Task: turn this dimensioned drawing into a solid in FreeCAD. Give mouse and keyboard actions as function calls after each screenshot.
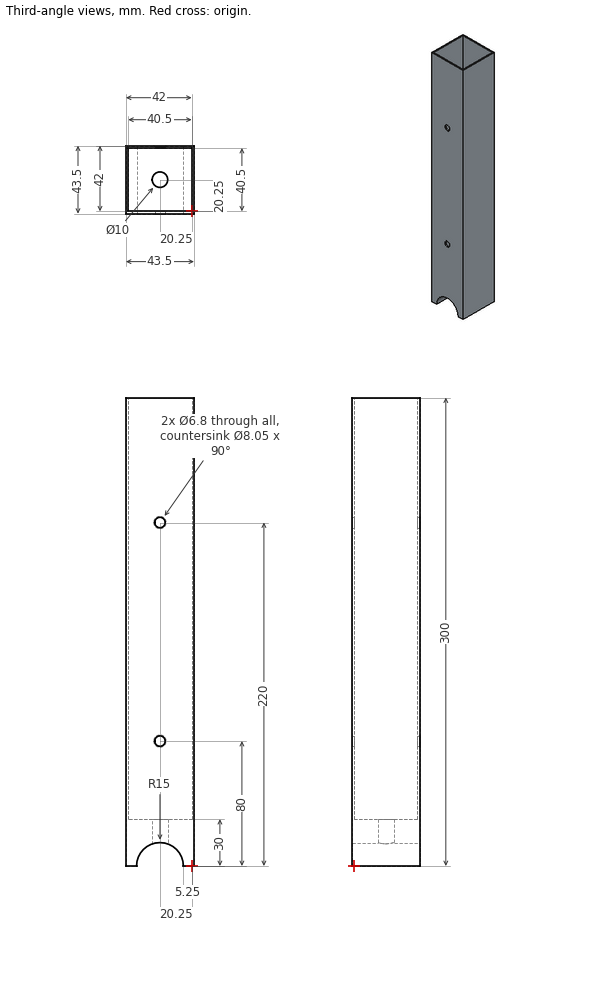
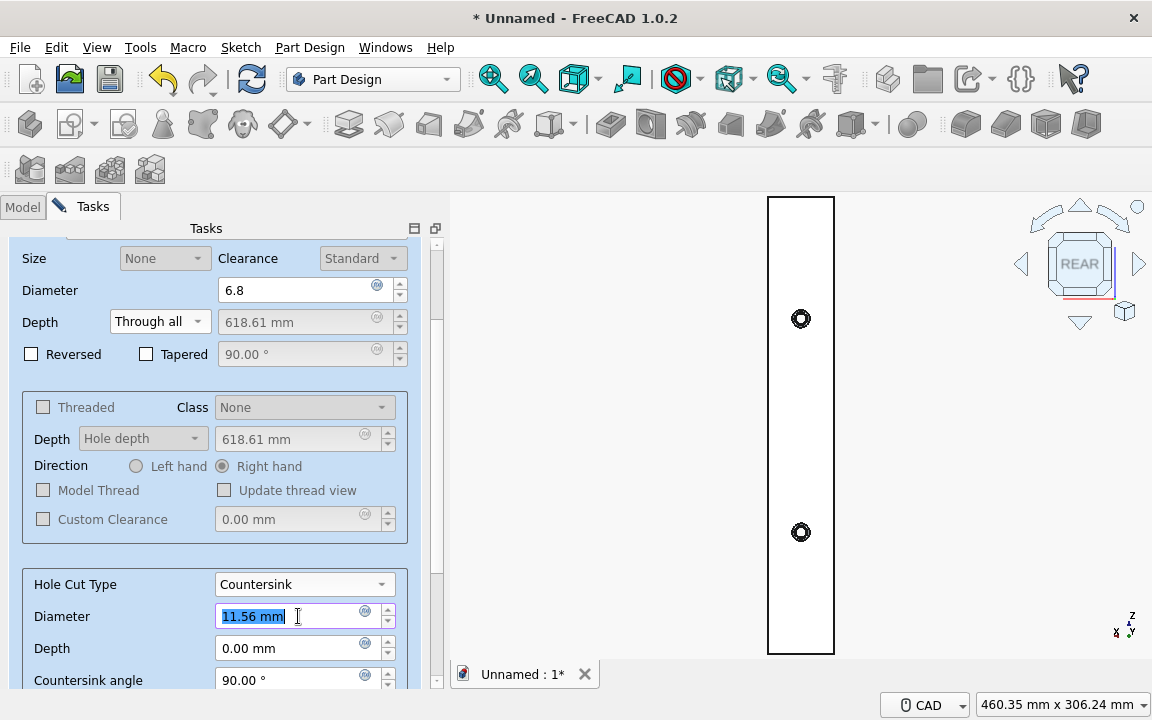
text(8.05)
key(Tab)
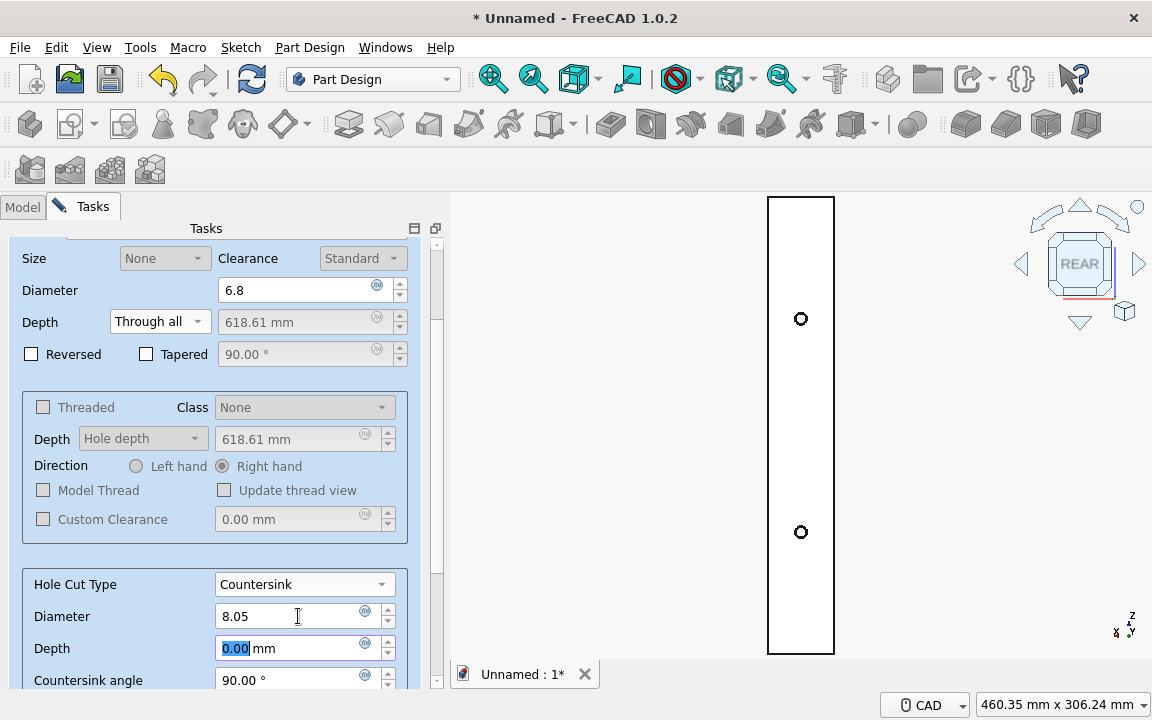
scroll(437, 463, up, 3)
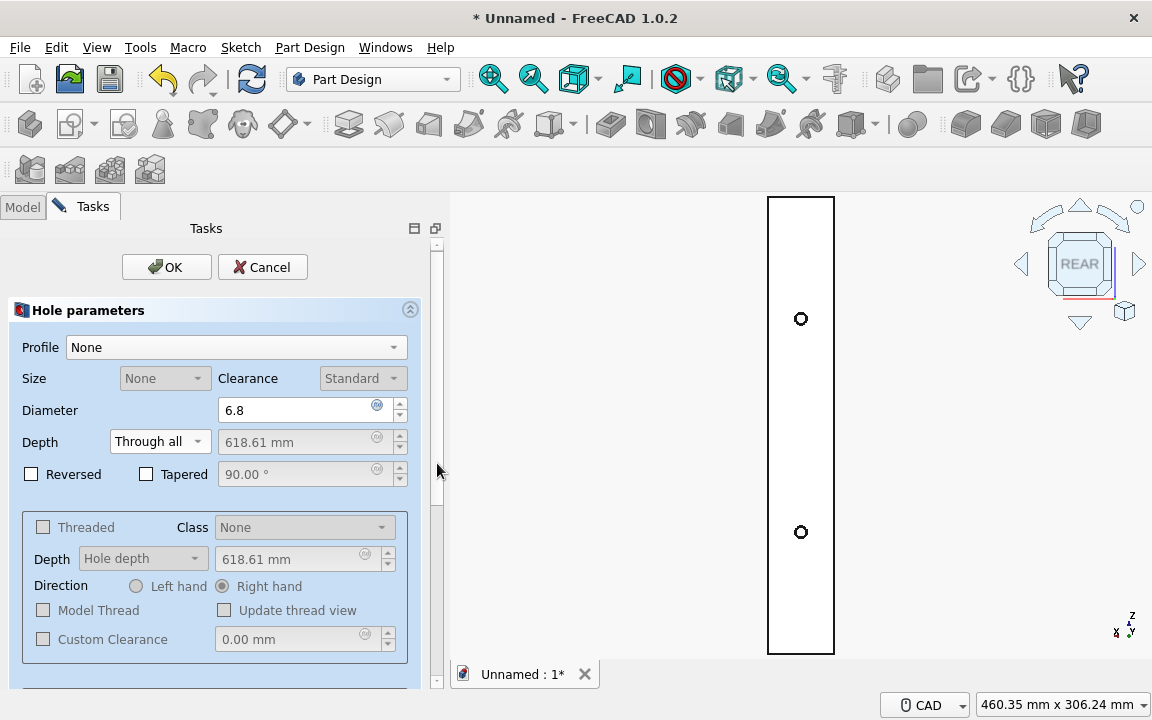
click(167, 267)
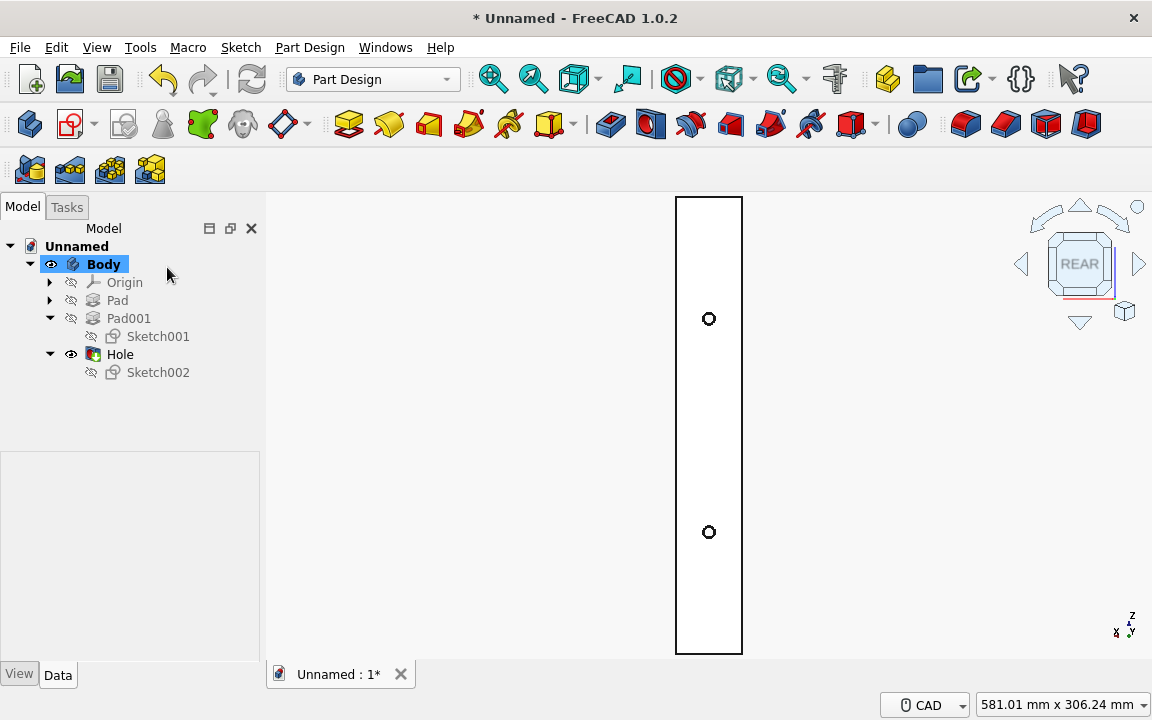
click(709, 359)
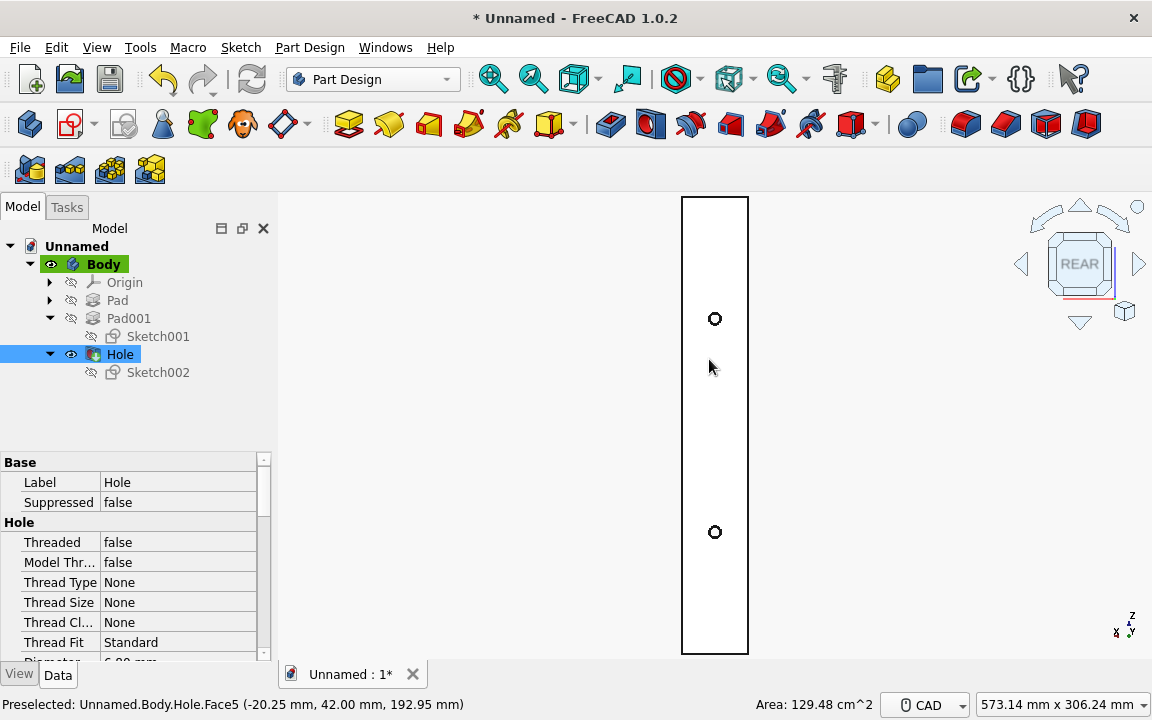
click(70, 124)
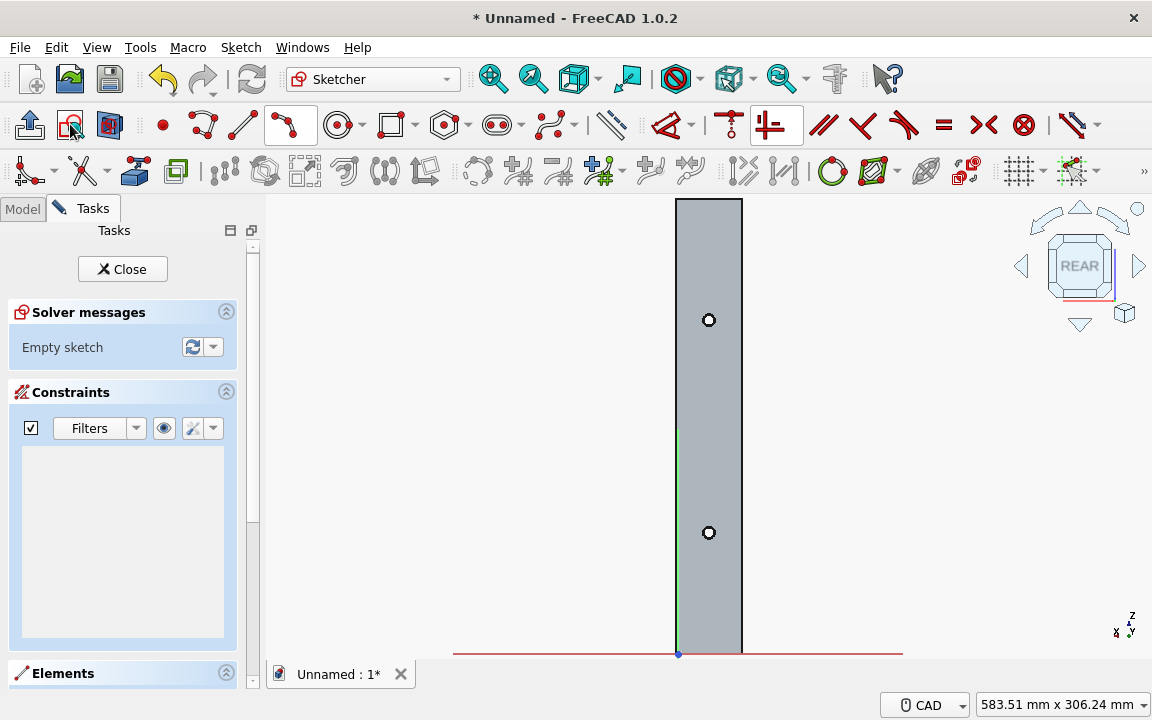
scroll(640, 426, down, 5)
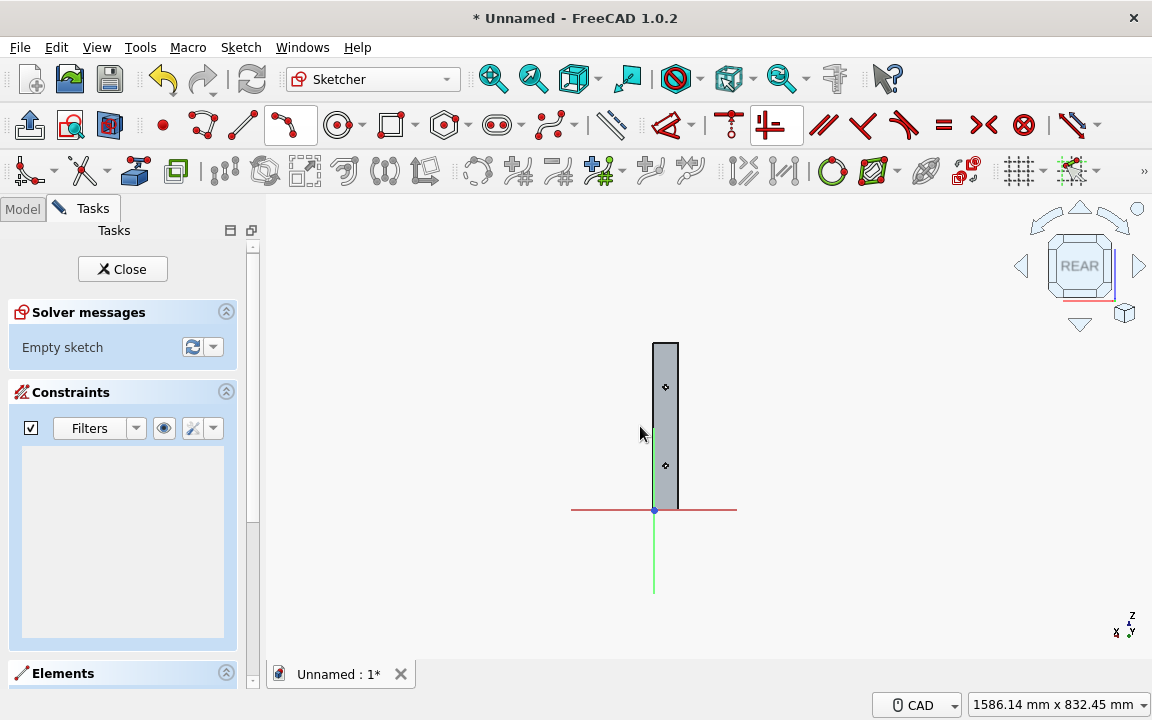
scroll(665, 510, up, 15)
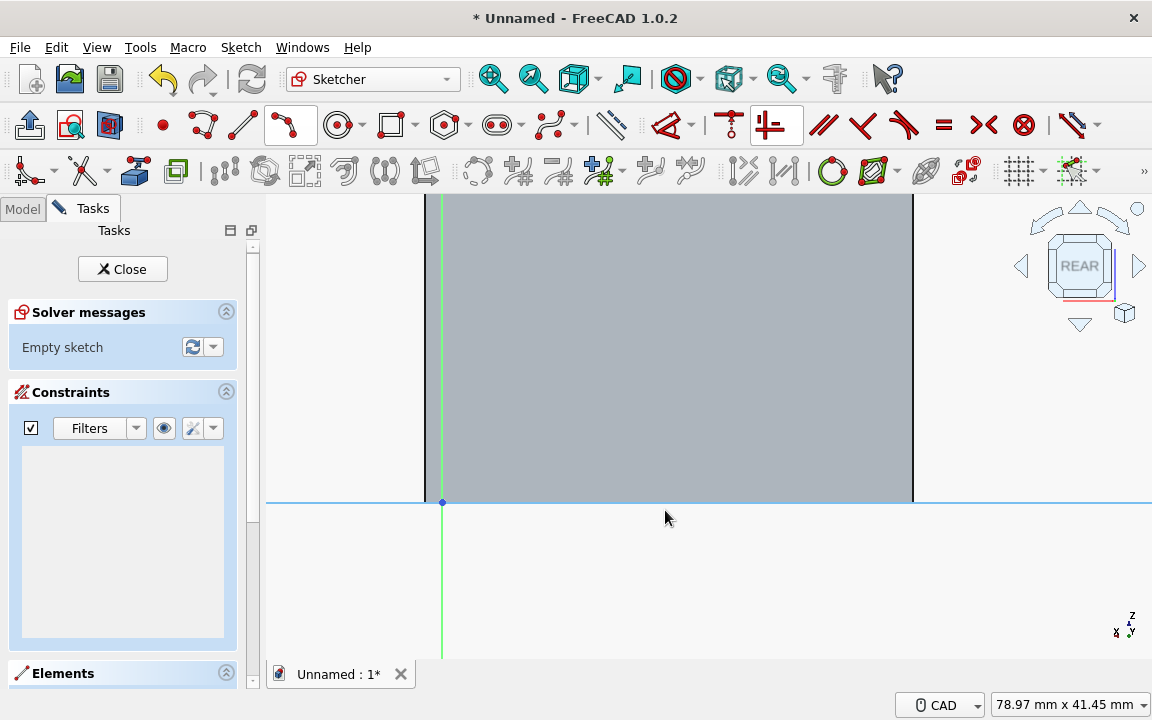
click(244, 126)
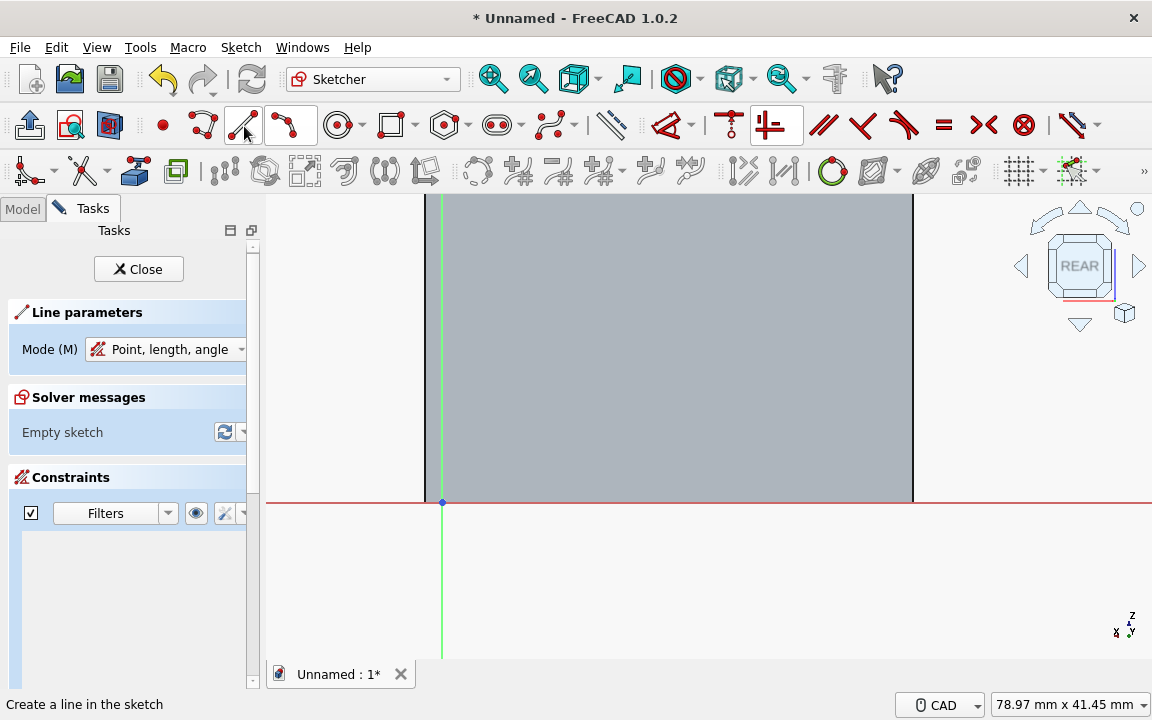
click(501, 503)
click(838, 494)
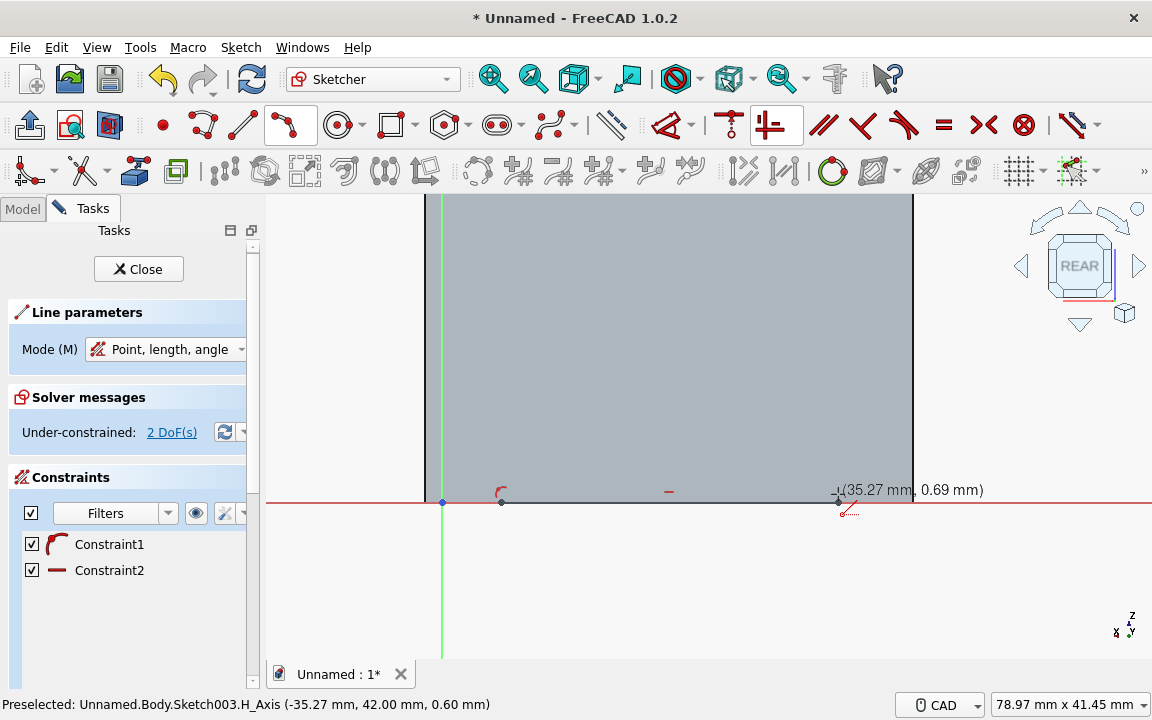
click(284, 126)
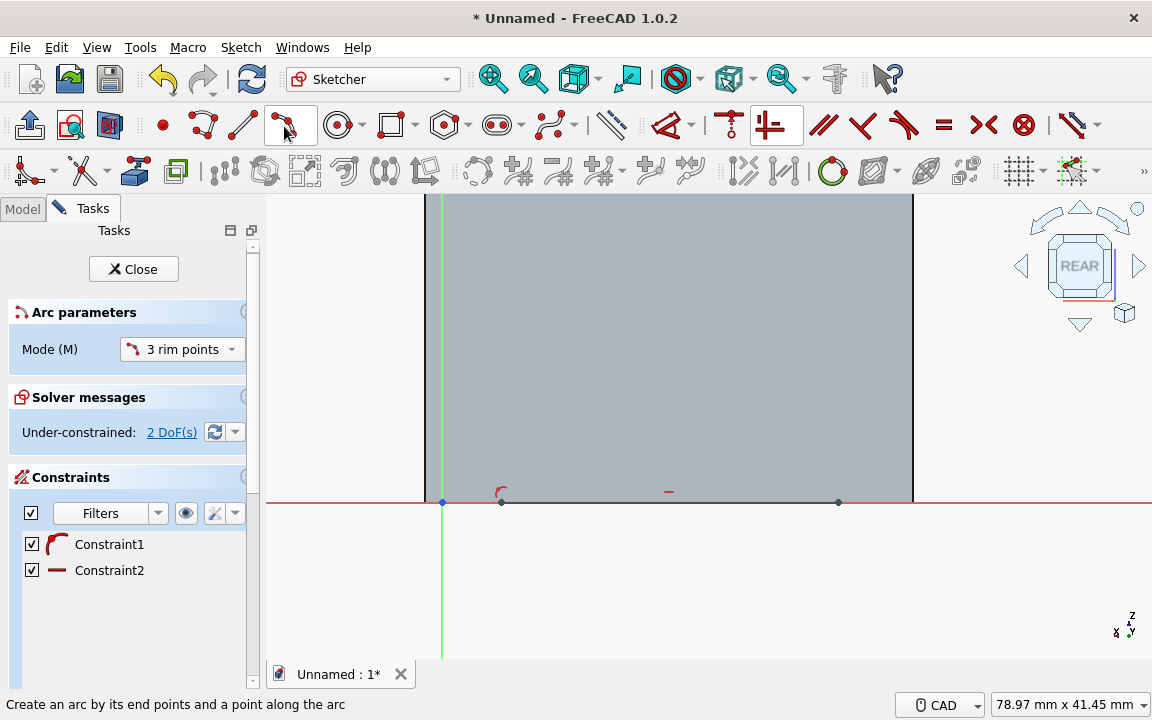
click(838, 503)
click(501, 503)
click(669, 335)
key(Escape)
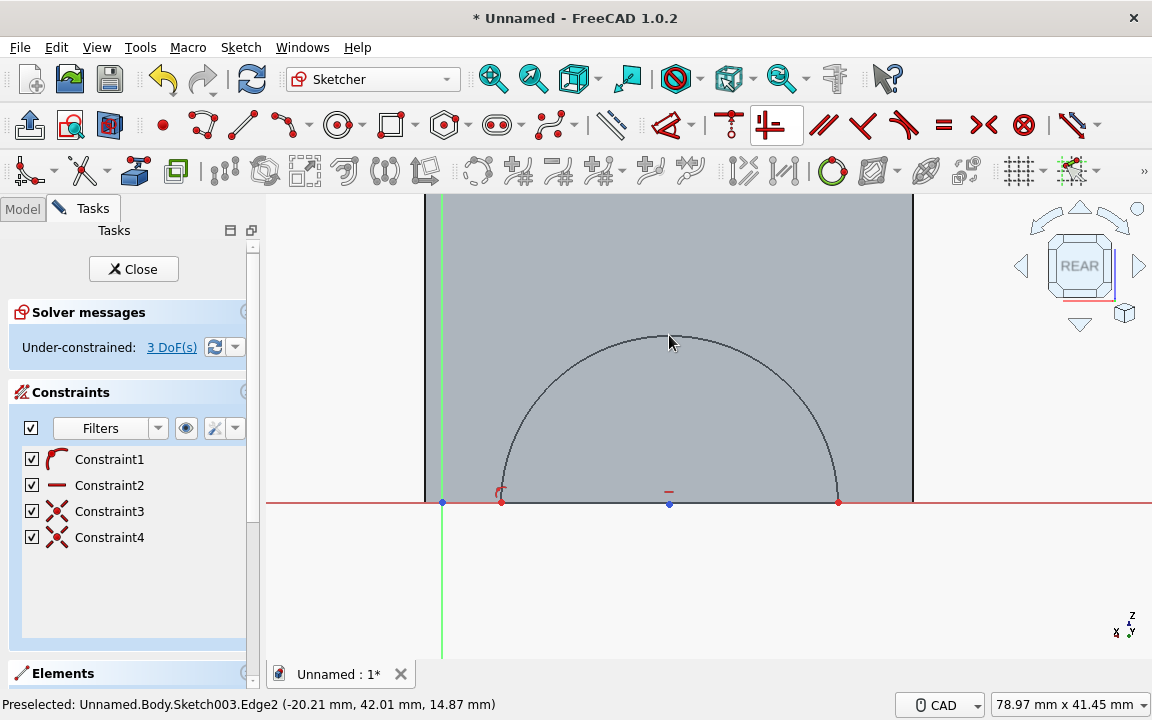
click(670, 505)